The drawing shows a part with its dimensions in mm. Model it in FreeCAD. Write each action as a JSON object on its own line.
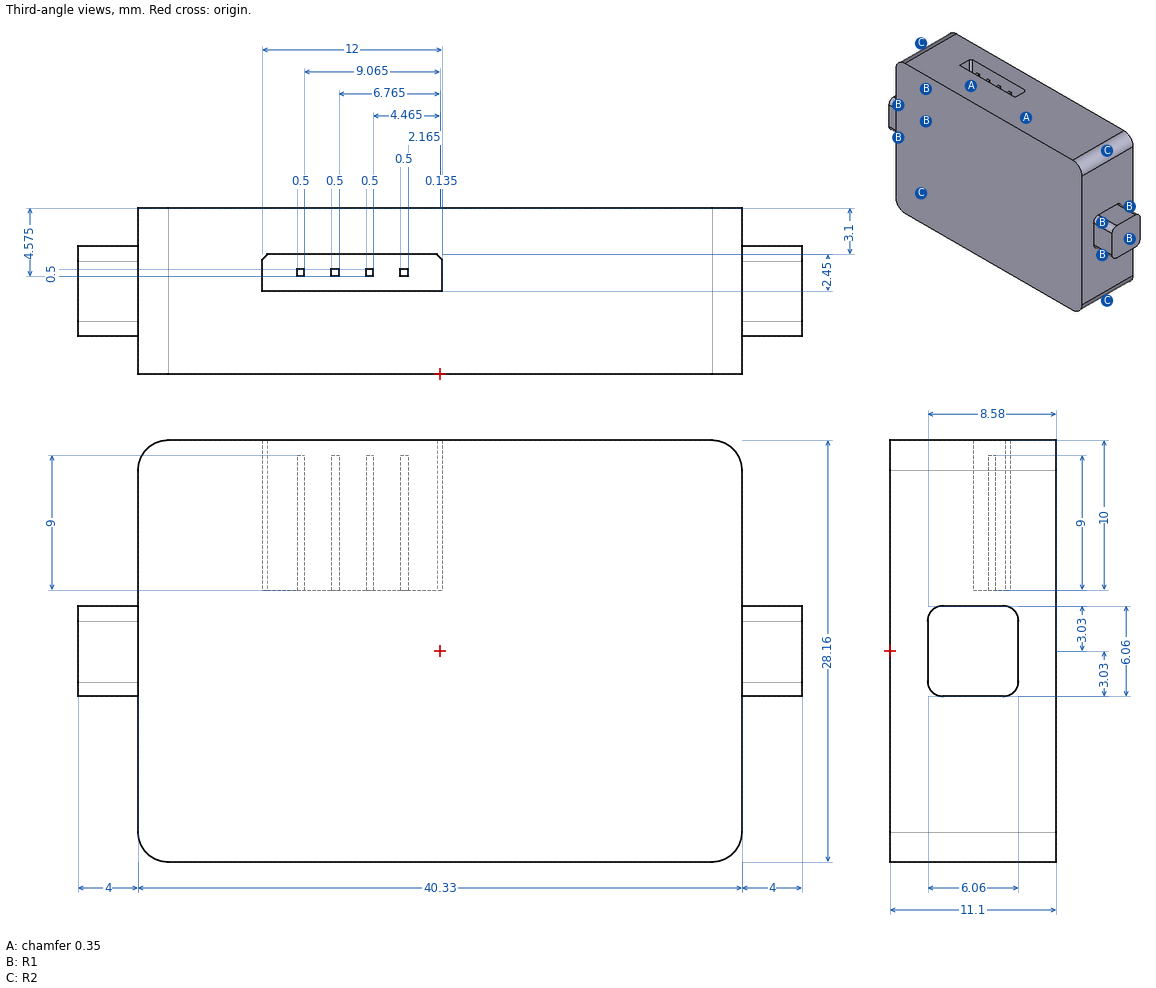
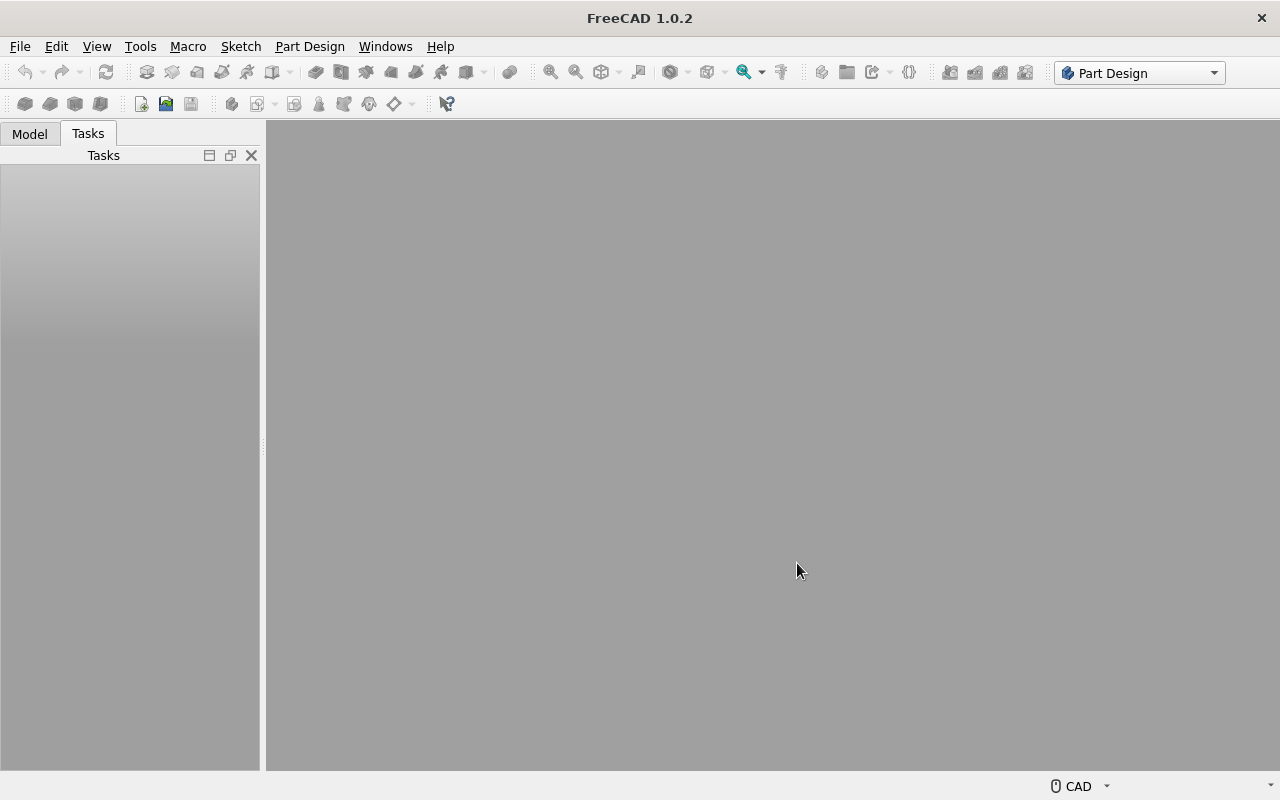
{"action": "key", "text": "ctrl+n"}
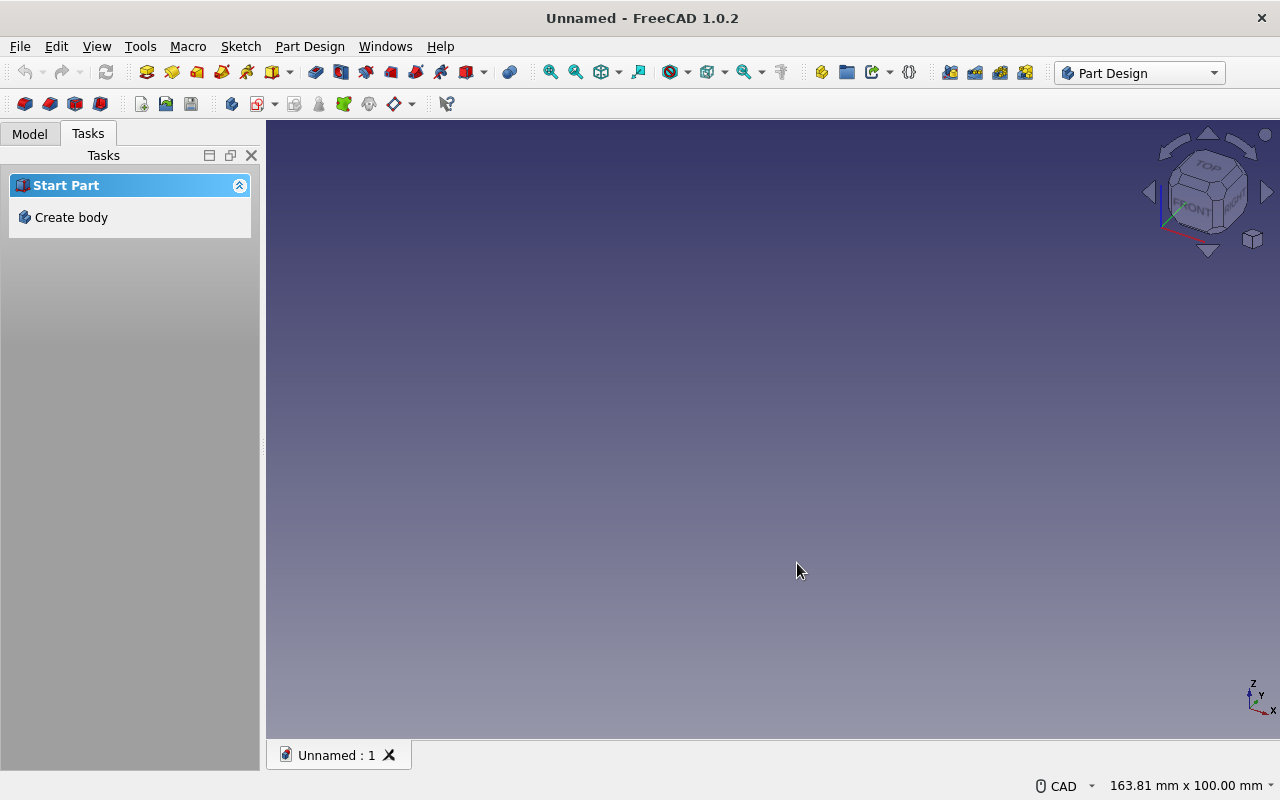
{"action": "left_click", "coordinate": [232, 104]}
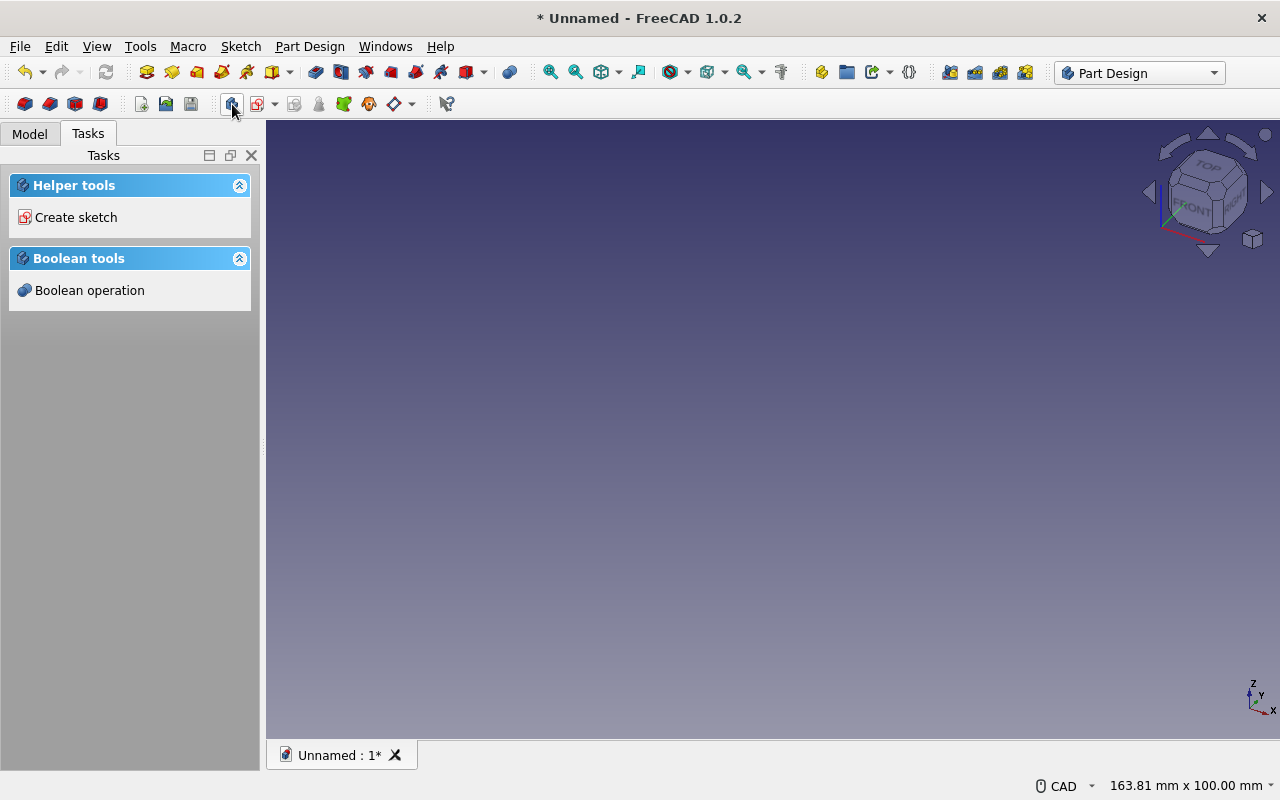
{"action": "left_click", "coordinate": [30, 134]}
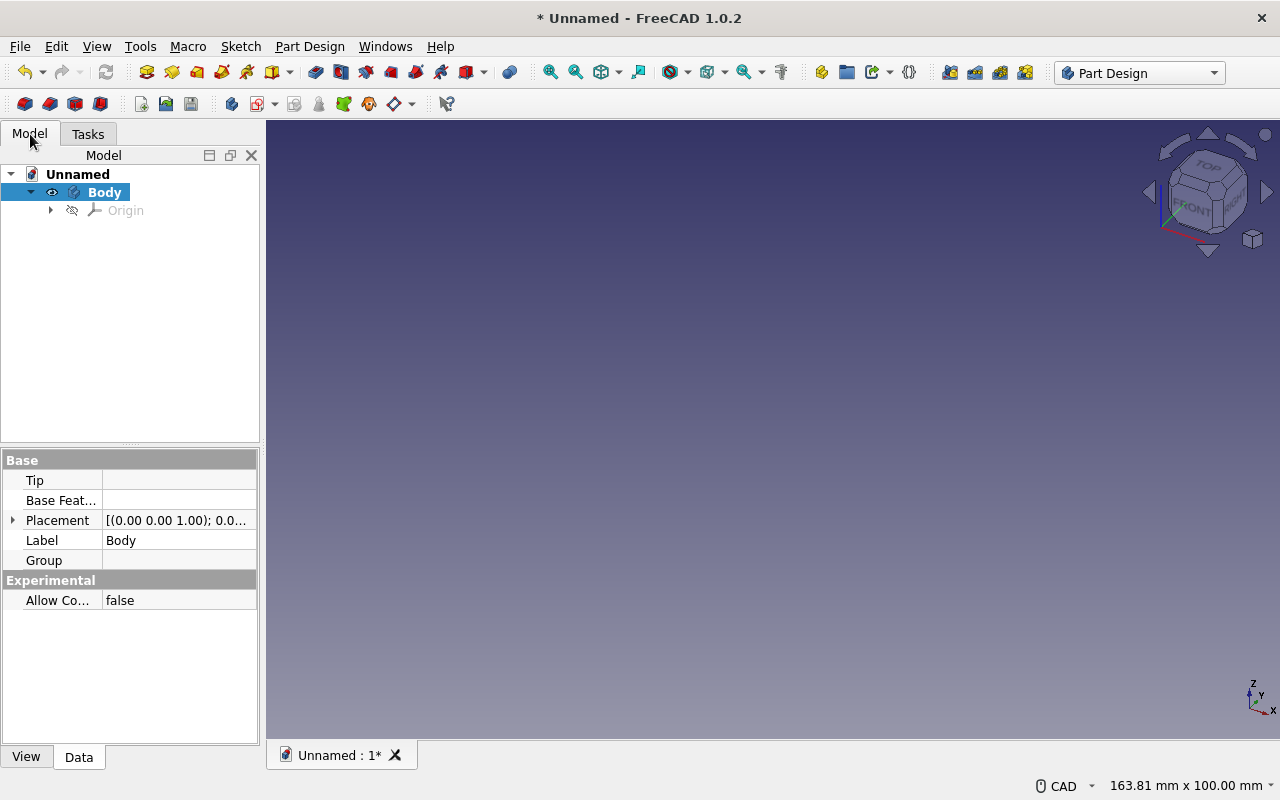
{"action": "left_click", "coordinate": [51, 210]}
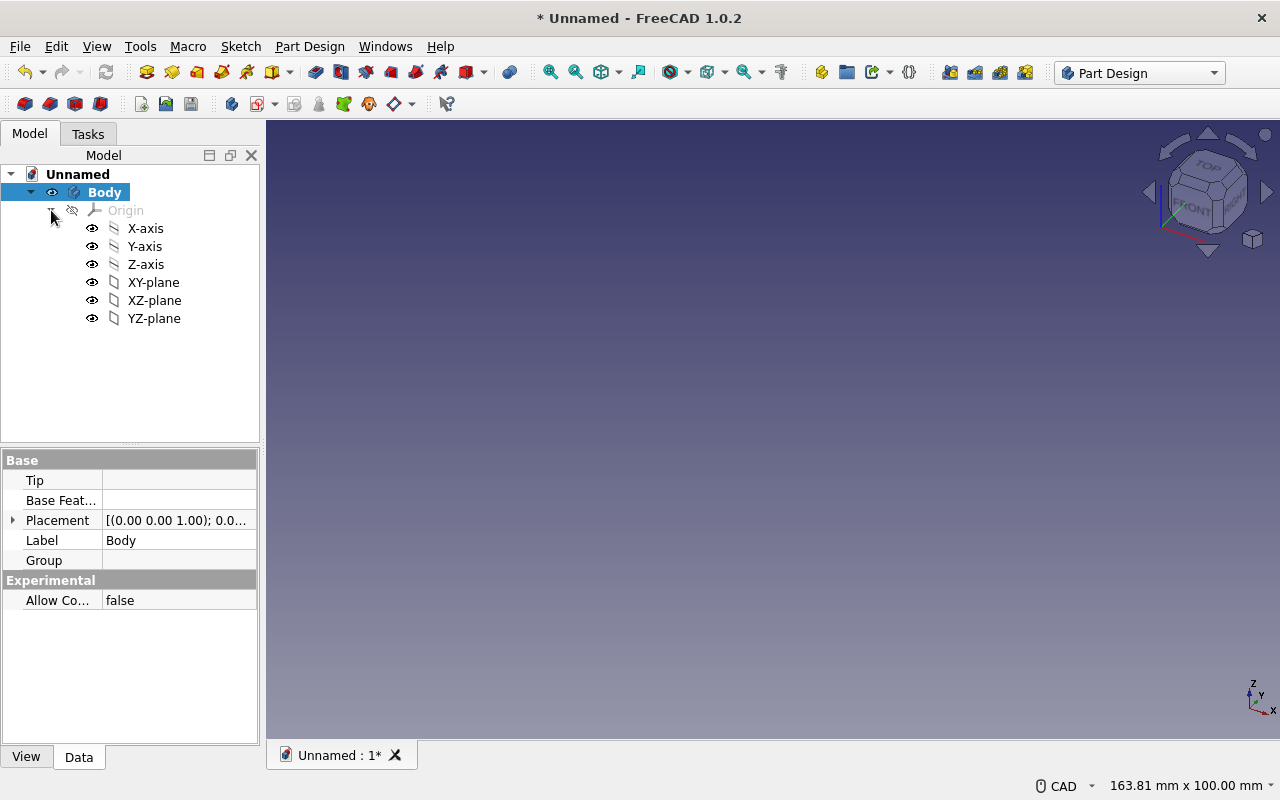
{"action": "left_click", "coordinate": [137, 300]}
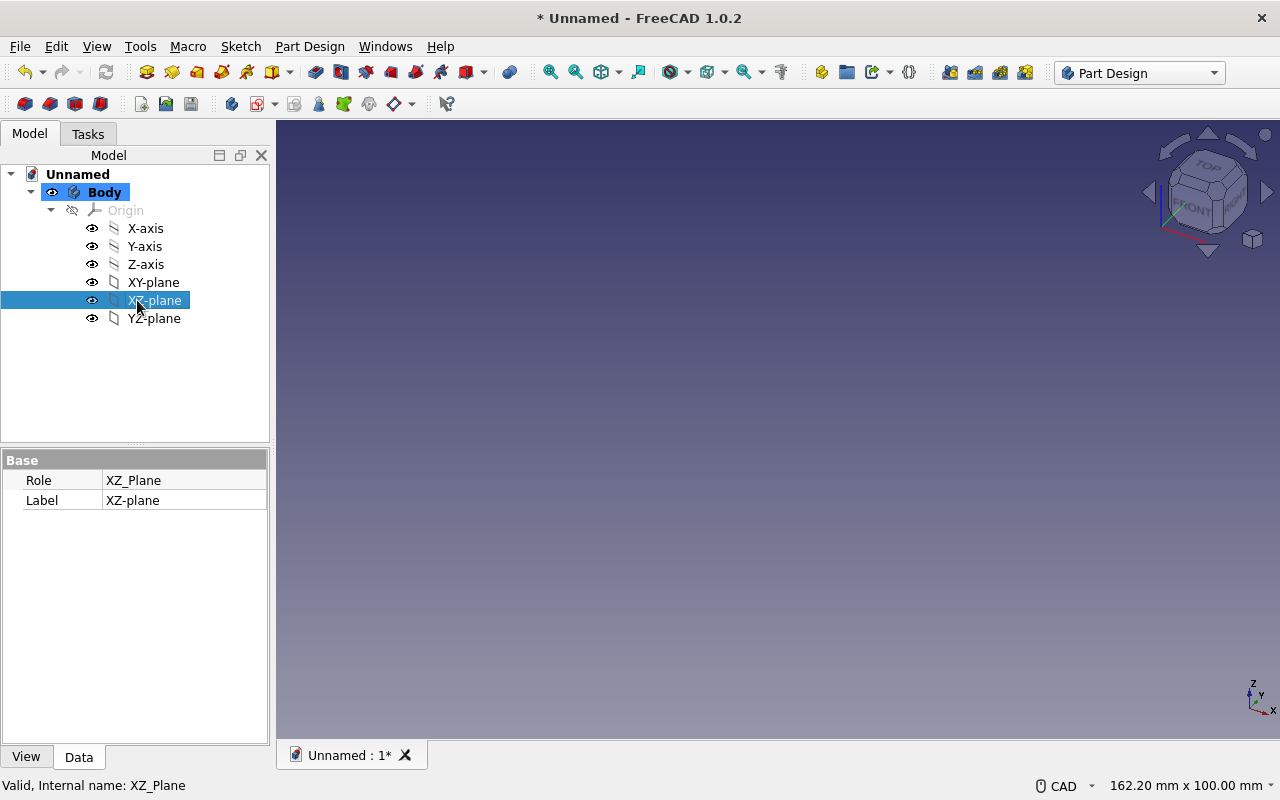
{"action": "left_click", "coordinate": [394, 104]}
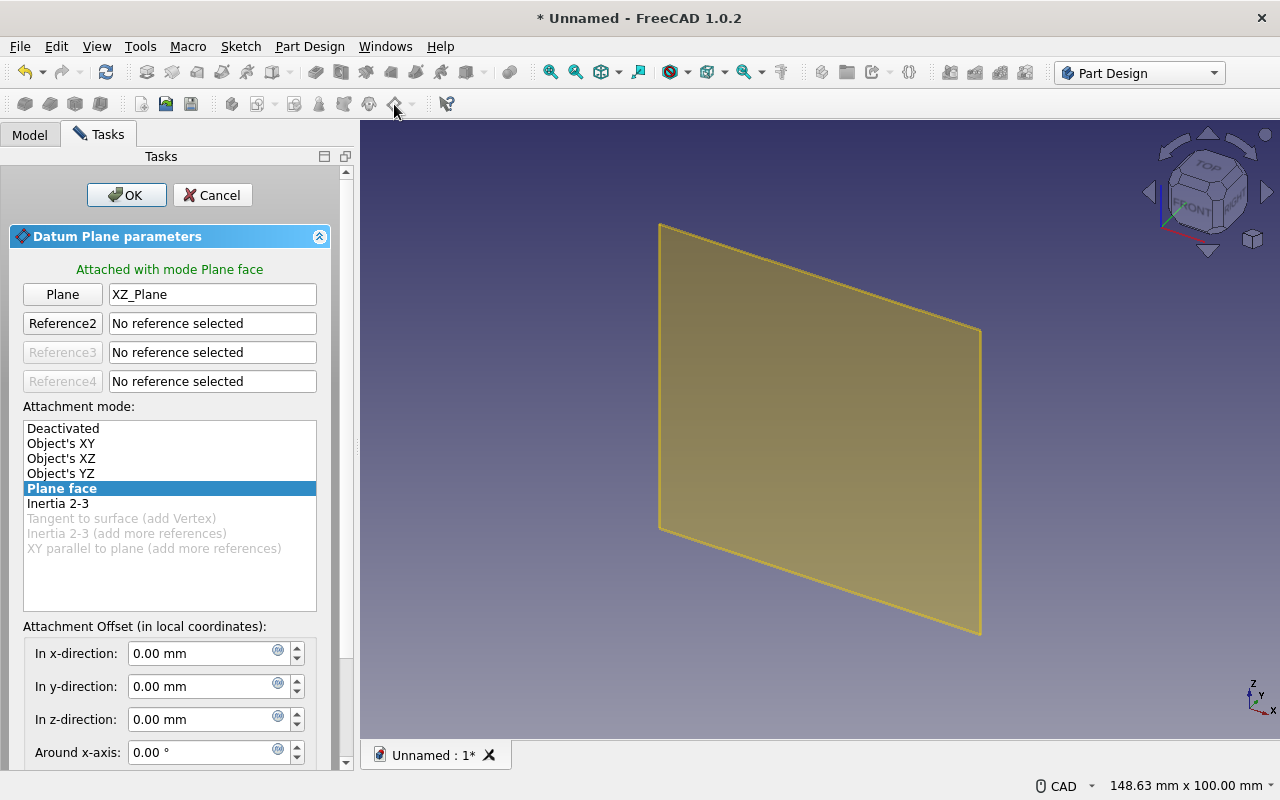
{"action": "triple_click", "coordinate": [210, 720]}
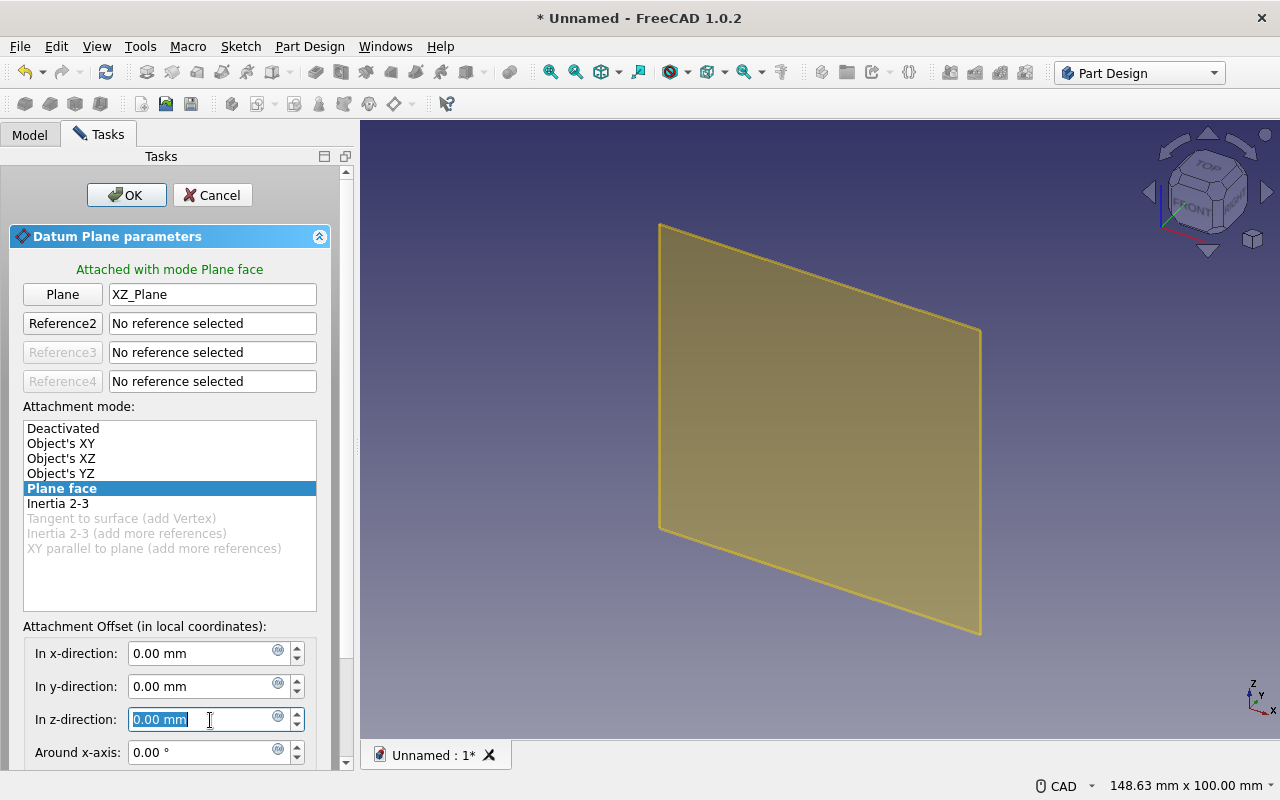
{"action": "type", "text": "-11.1"}
{"action": "key", "text": "Tab"}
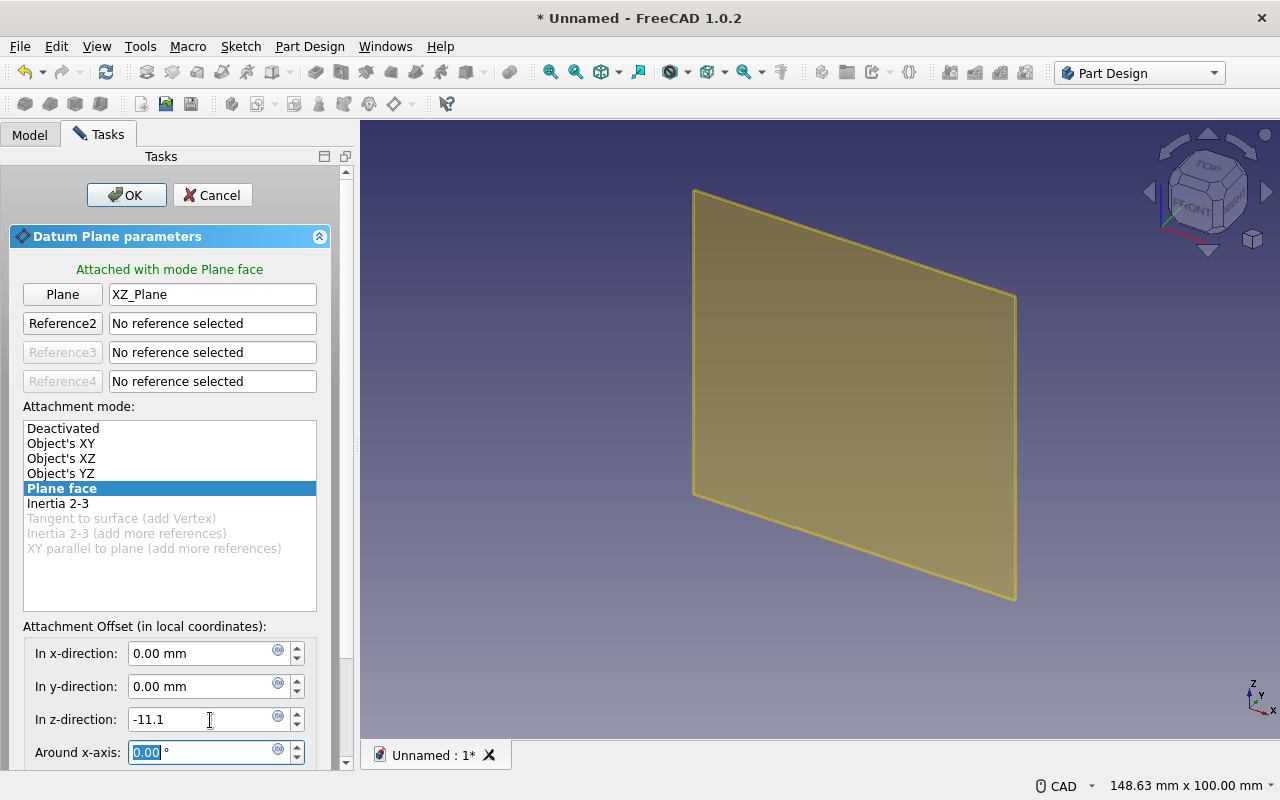
{"action": "left_click", "coordinate": [127, 195]}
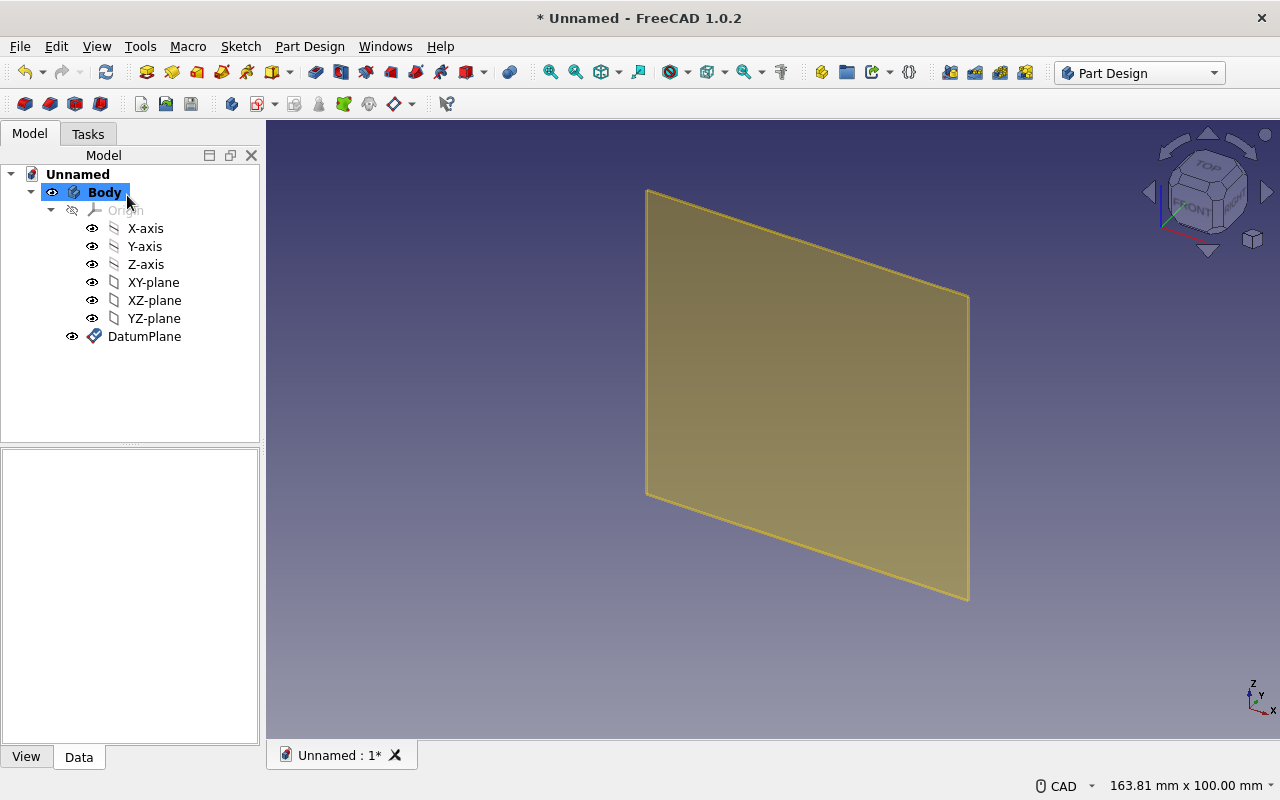
{"action": "left_click", "coordinate": [117, 336]}